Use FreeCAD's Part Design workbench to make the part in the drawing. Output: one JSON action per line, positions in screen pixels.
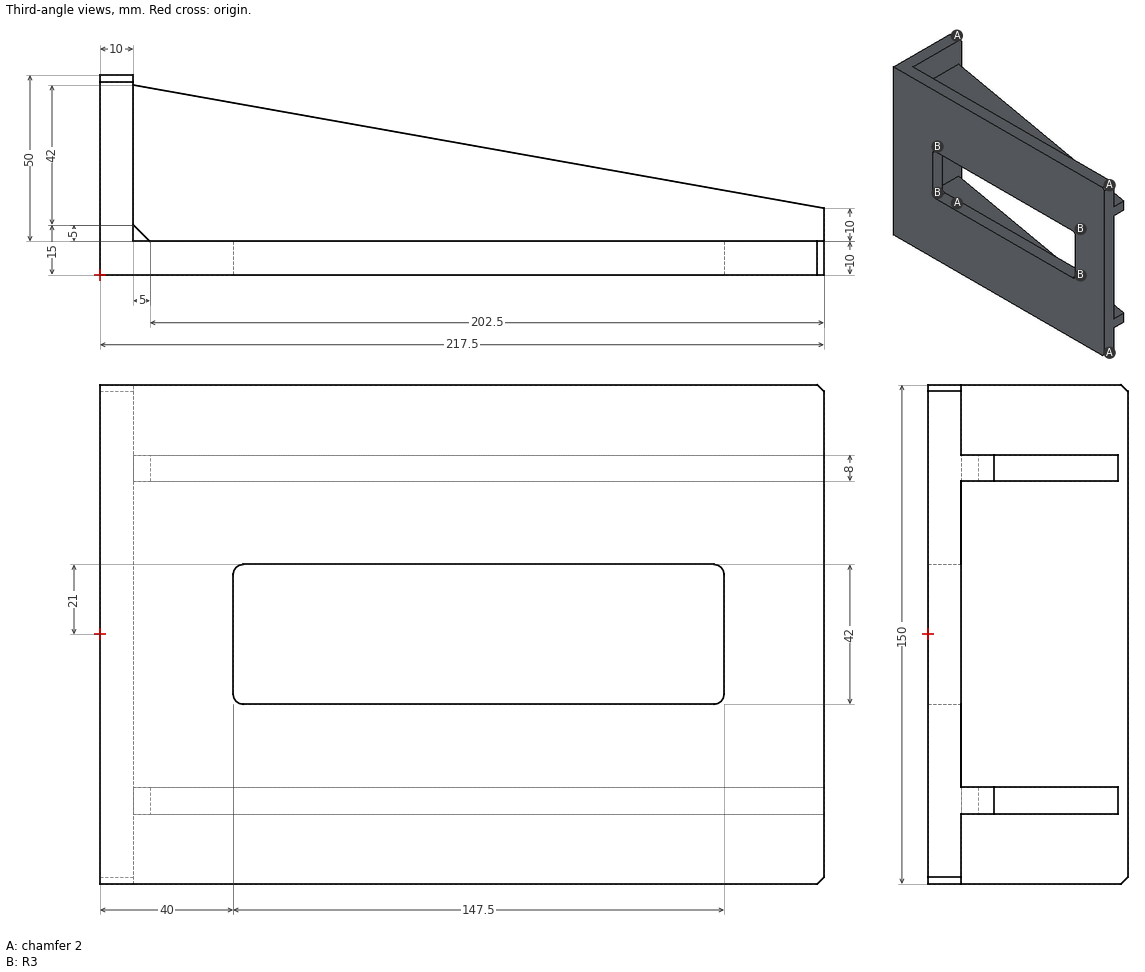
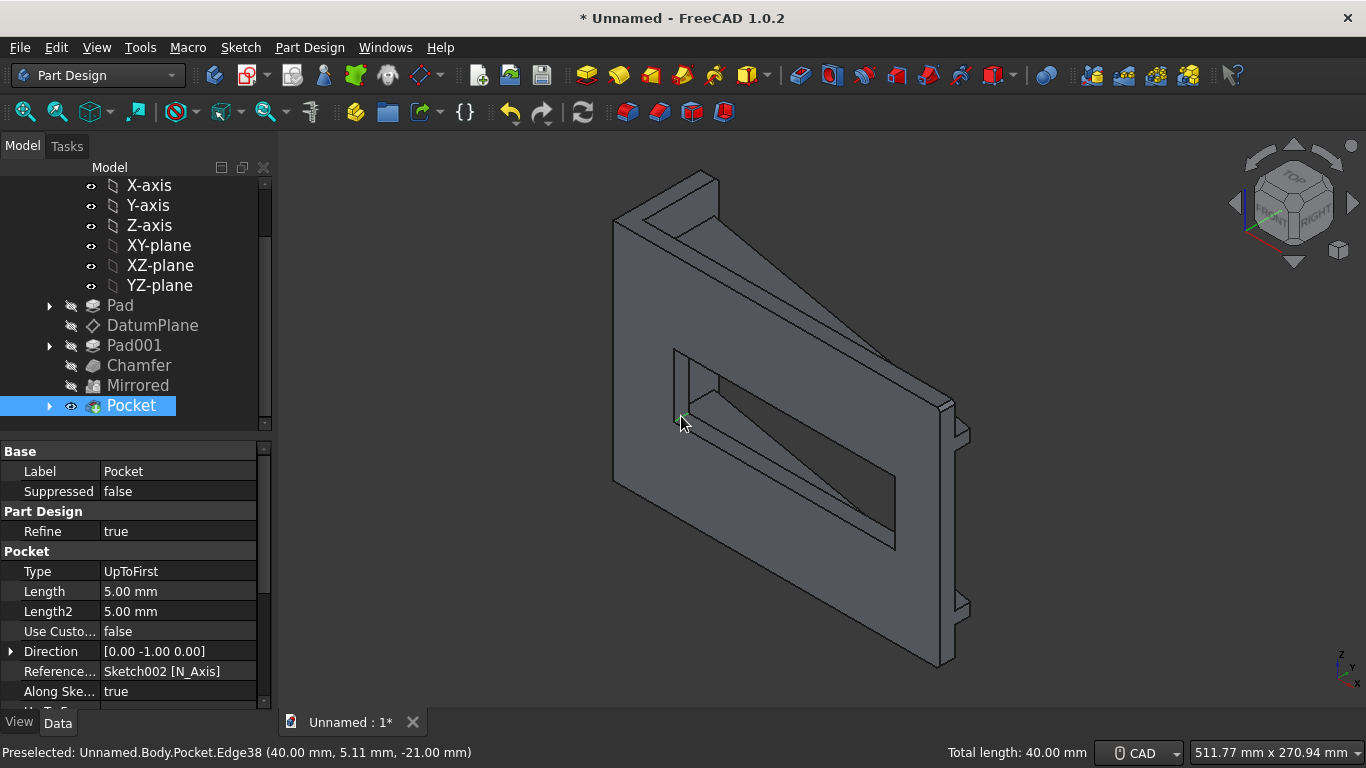
{"action": "left_click", "coordinate": [628, 112]}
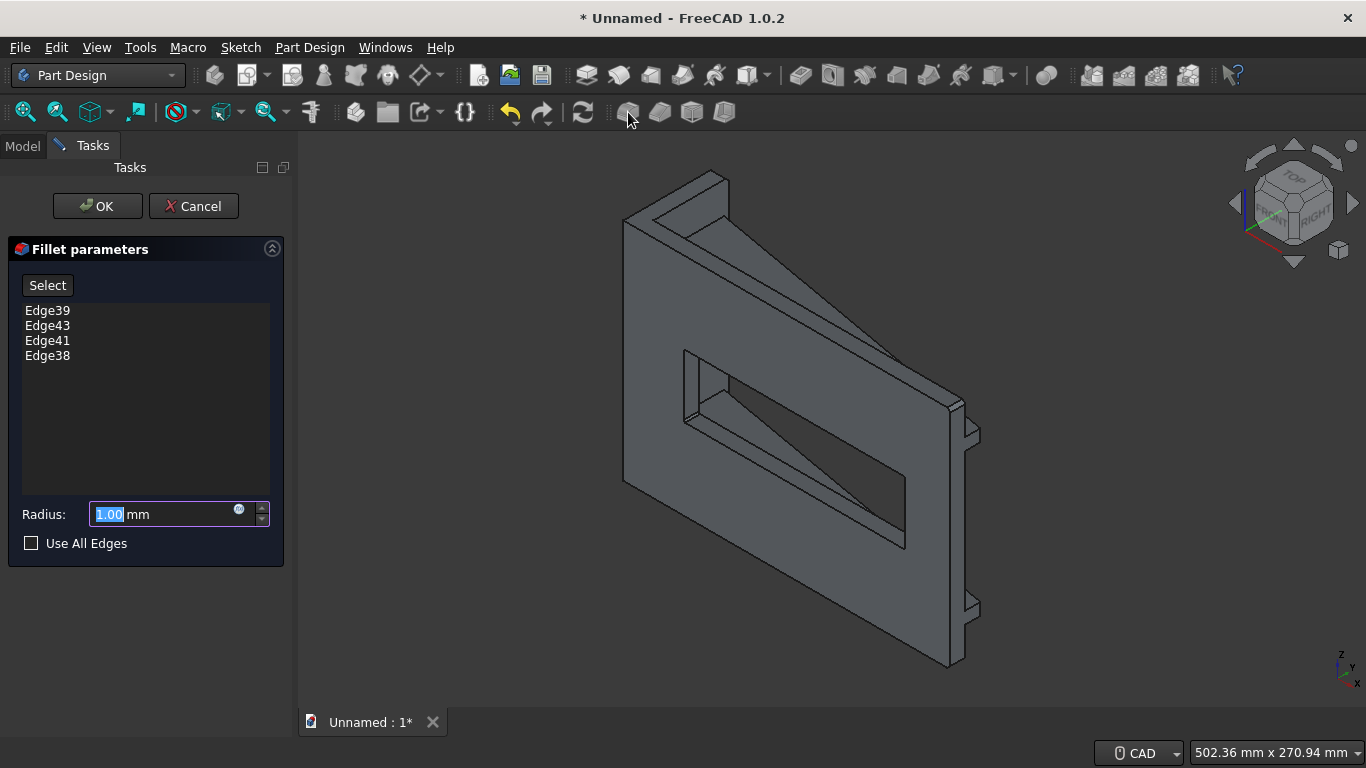
{"action": "type", "text": "3"}
{"action": "key", "text": "Tab"}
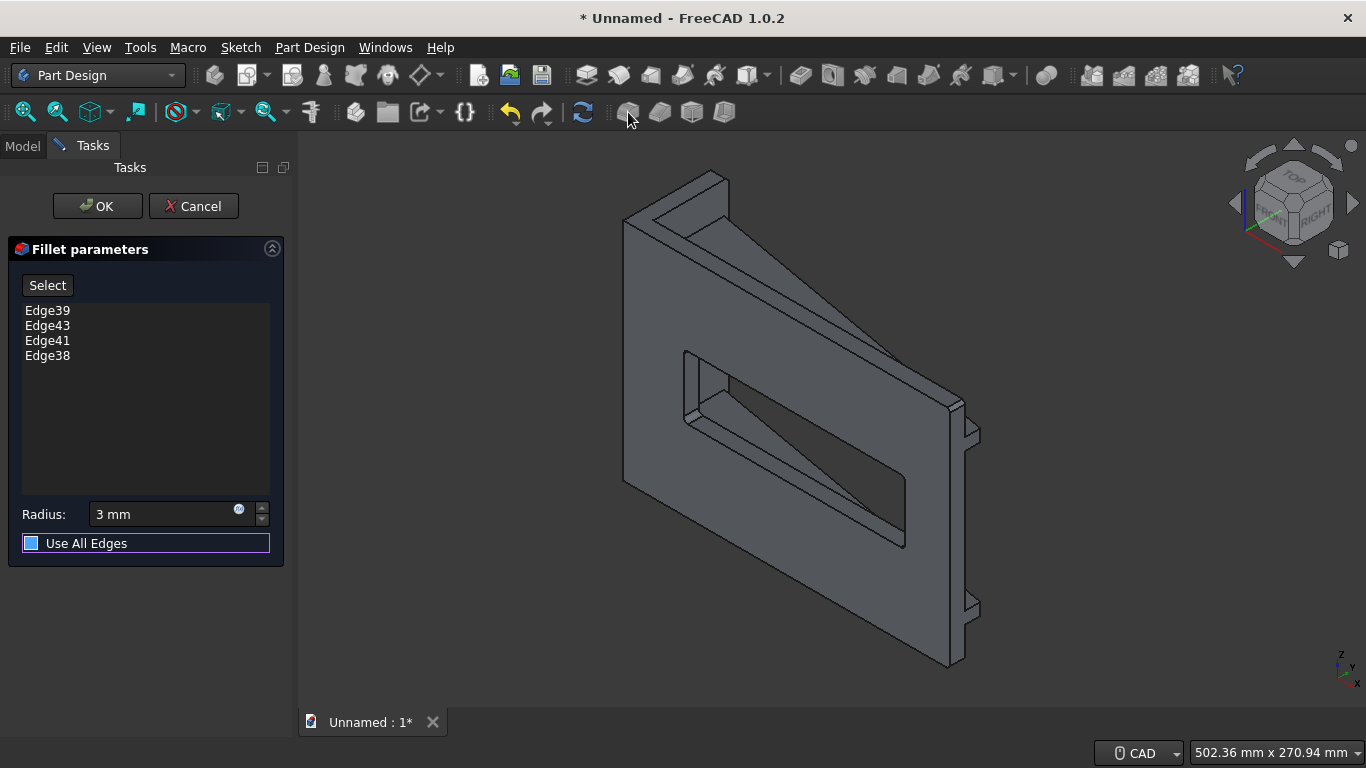
{"action": "left_click", "coordinate": [98, 206]}